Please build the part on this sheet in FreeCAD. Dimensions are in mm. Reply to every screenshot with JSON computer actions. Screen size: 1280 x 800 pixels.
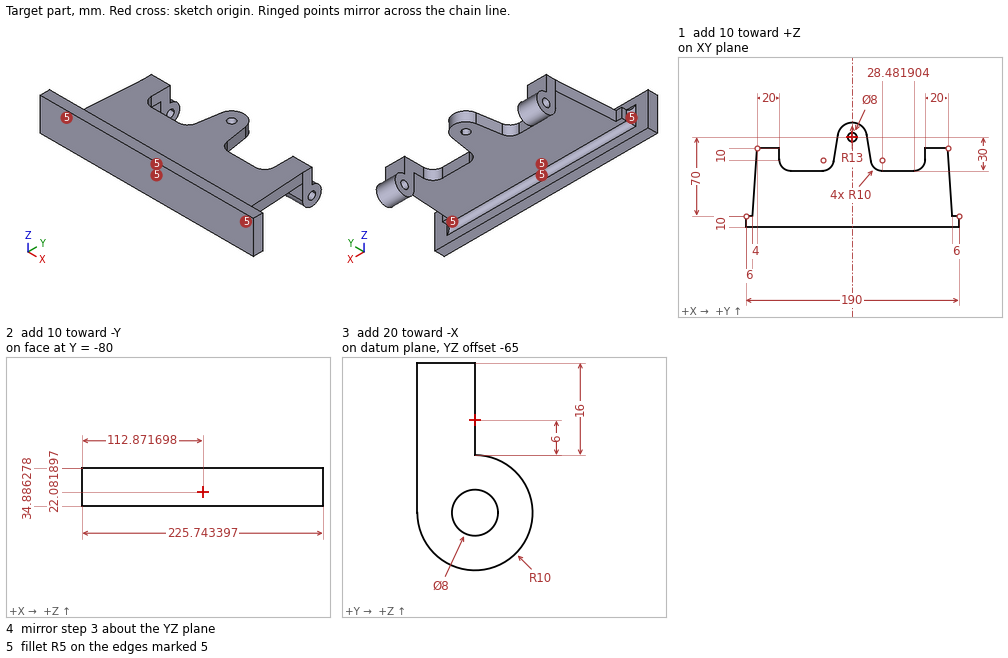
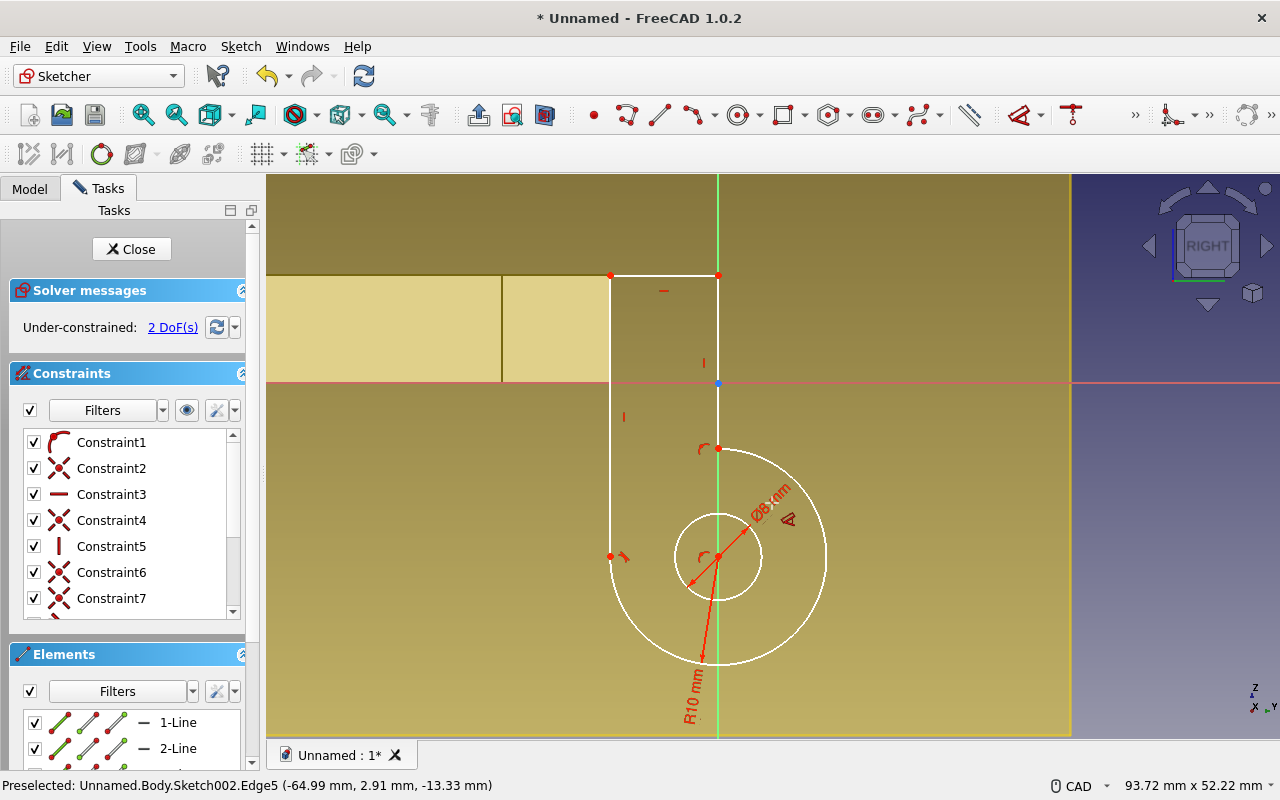
{"action": "left_click", "coordinate": [718, 397]}
{"action": "left_click", "coordinate": [752, 362]}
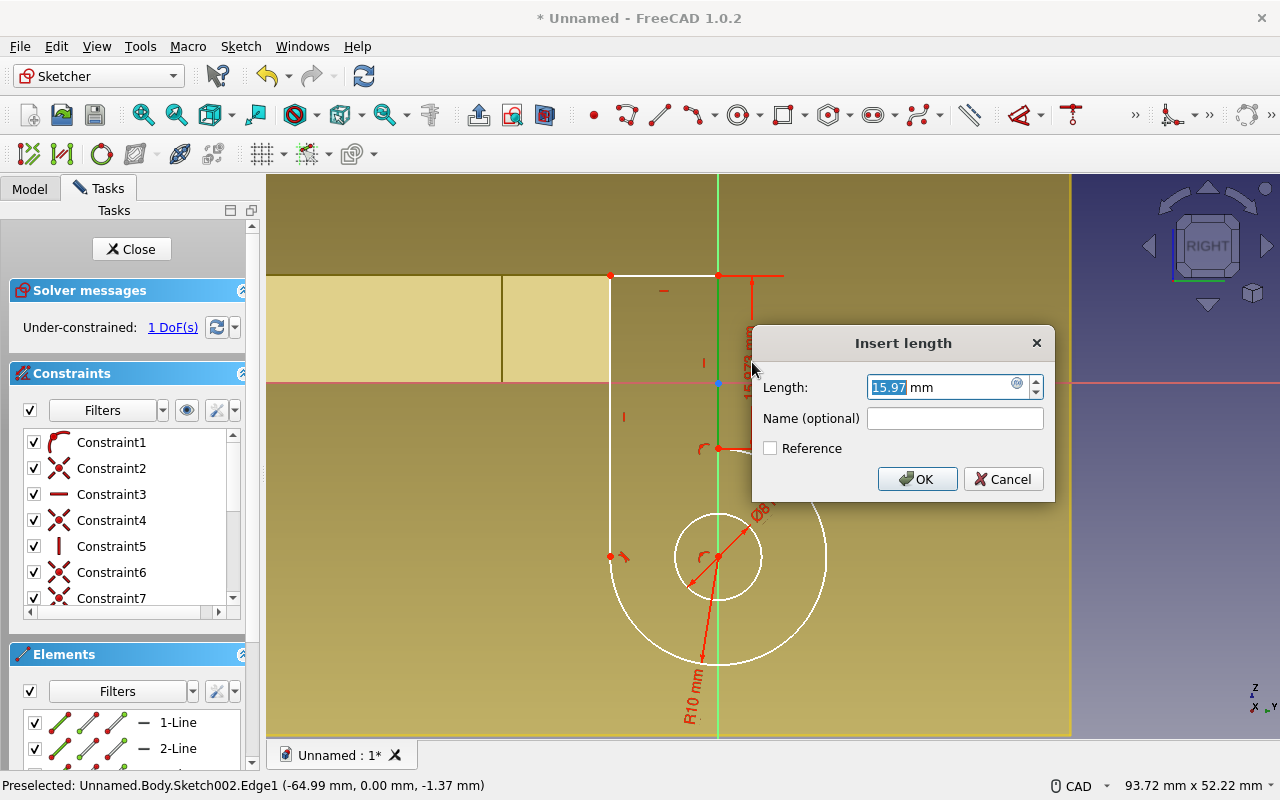
{"action": "type", "text": "16"}
{"action": "key", "text": "Return"}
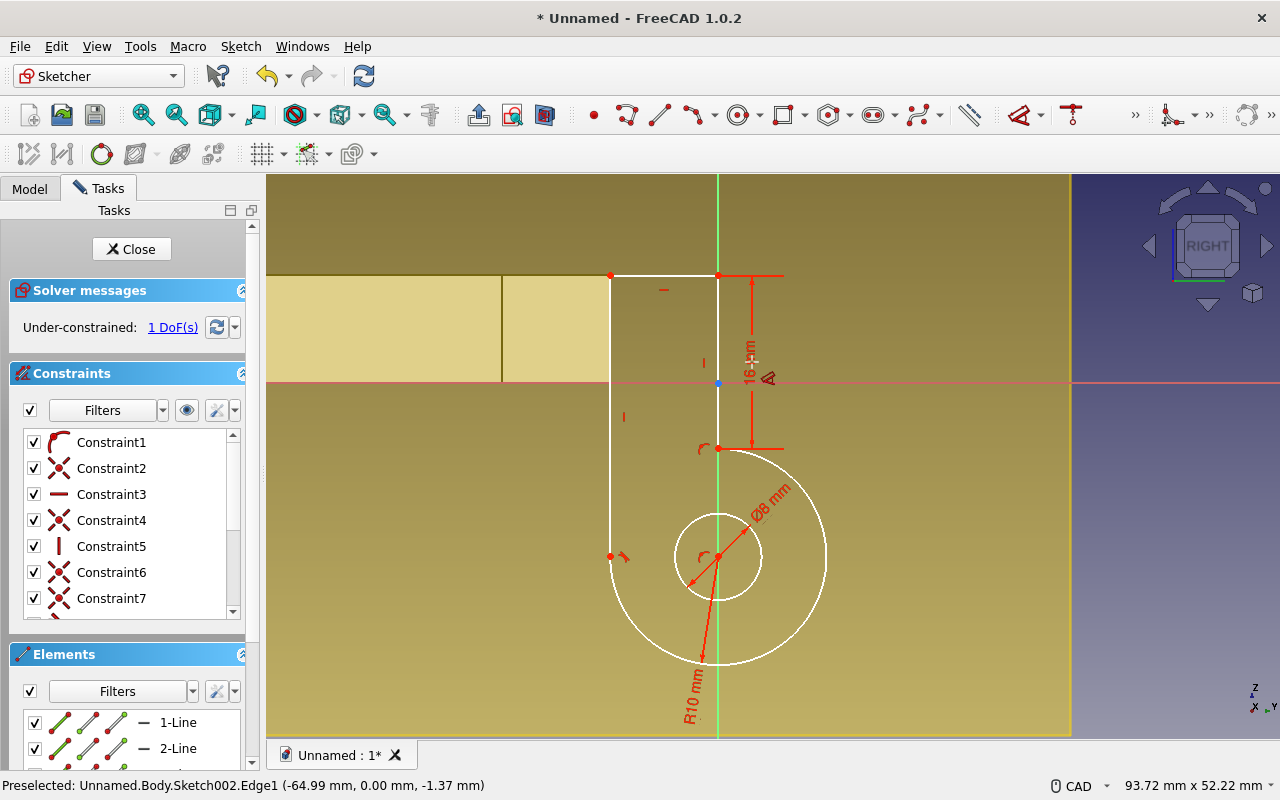
{"action": "left_click", "coordinate": [718, 449]}
{"action": "left_click", "coordinate": [752, 416]}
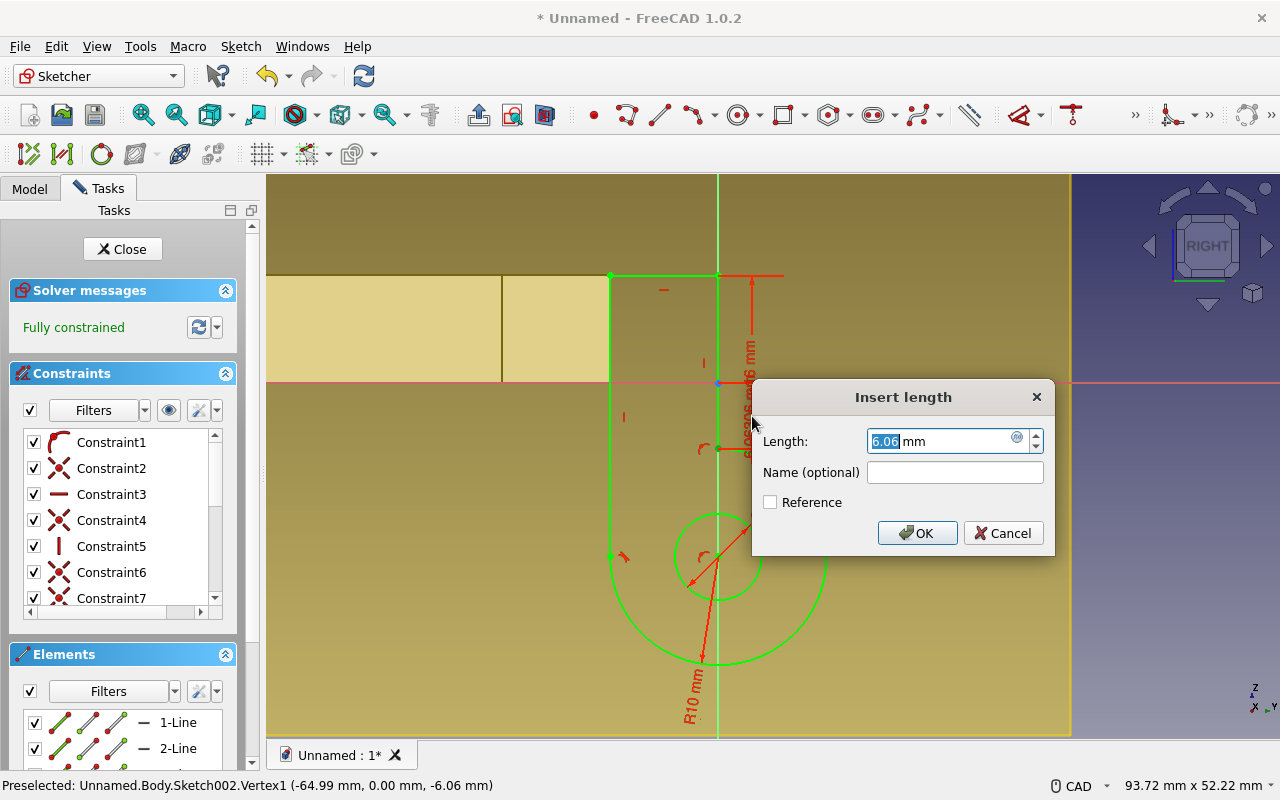
{"action": "type", "text": "6"}
{"action": "key", "text": "Return"}
{"action": "key", "text": "Escape"}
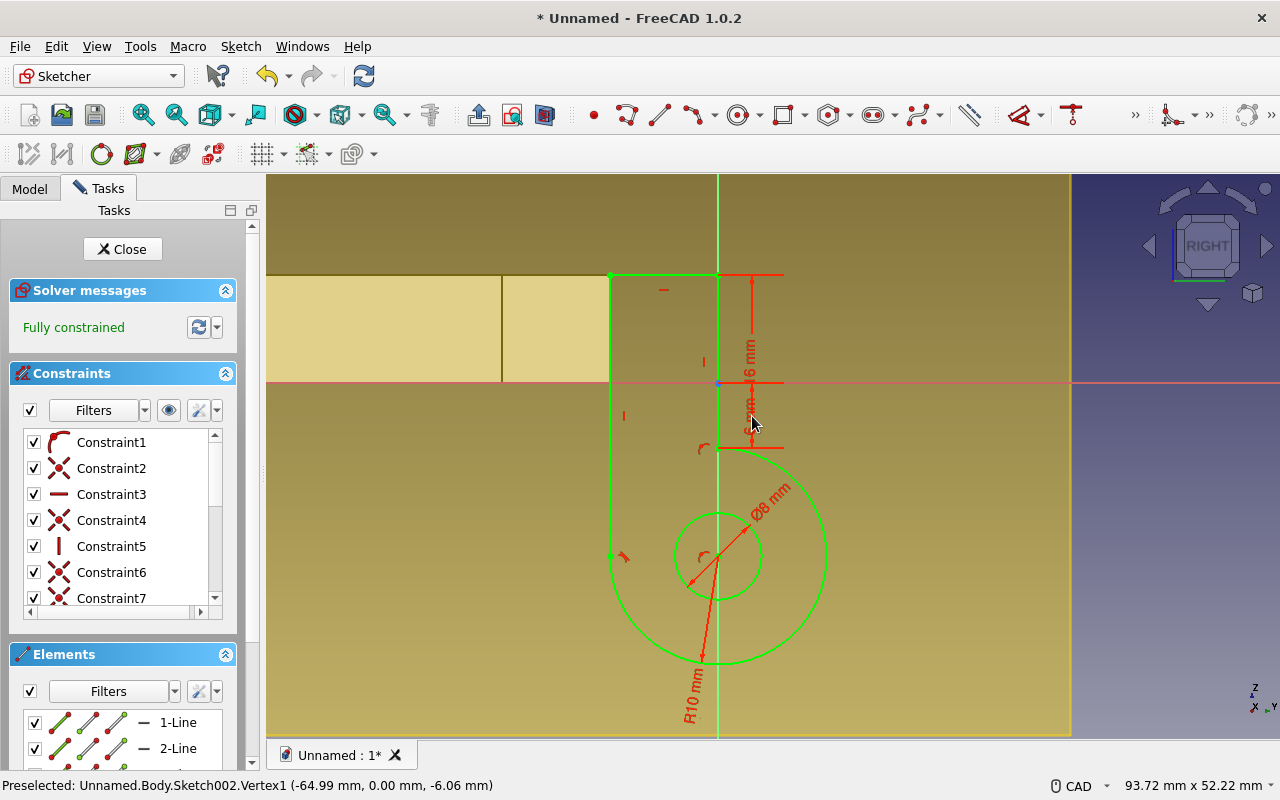
{"action": "left_click", "coordinate": [123, 249]}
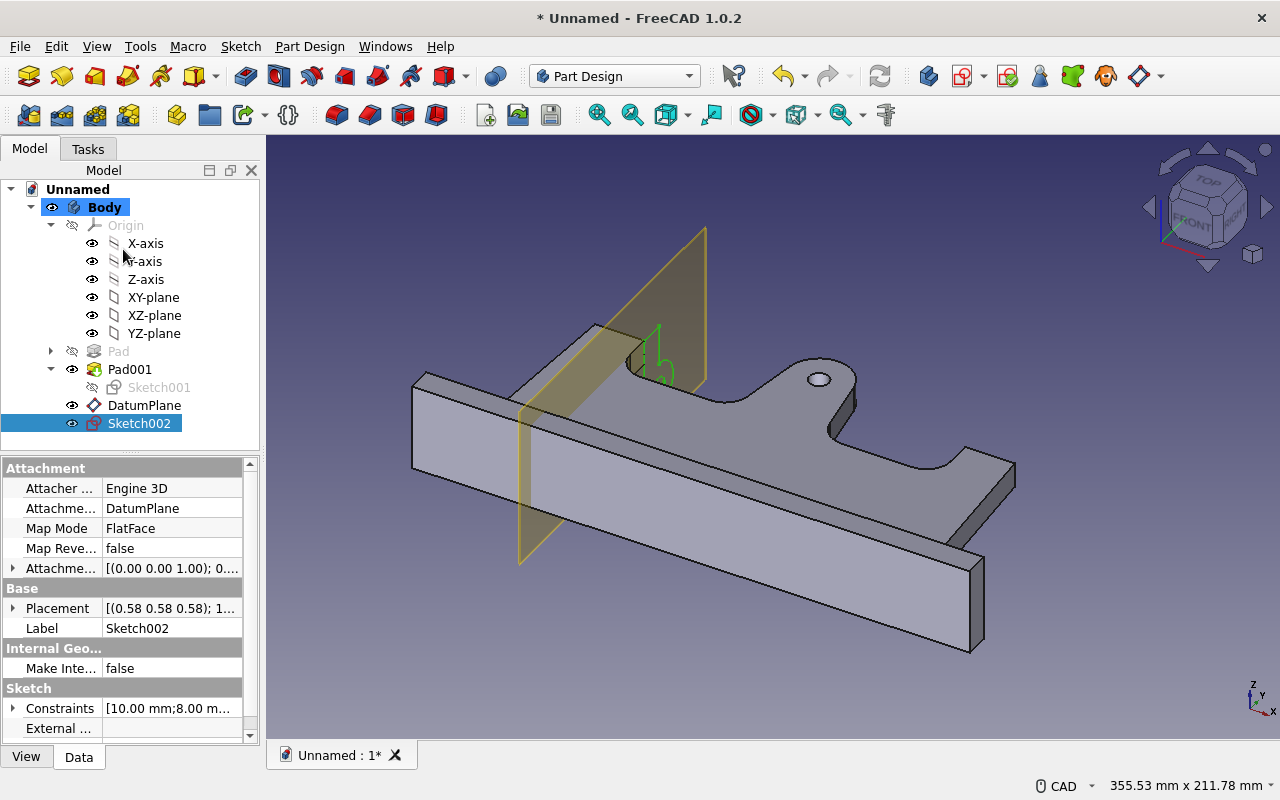
{"action": "left_click", "coordinate": [29, 76]}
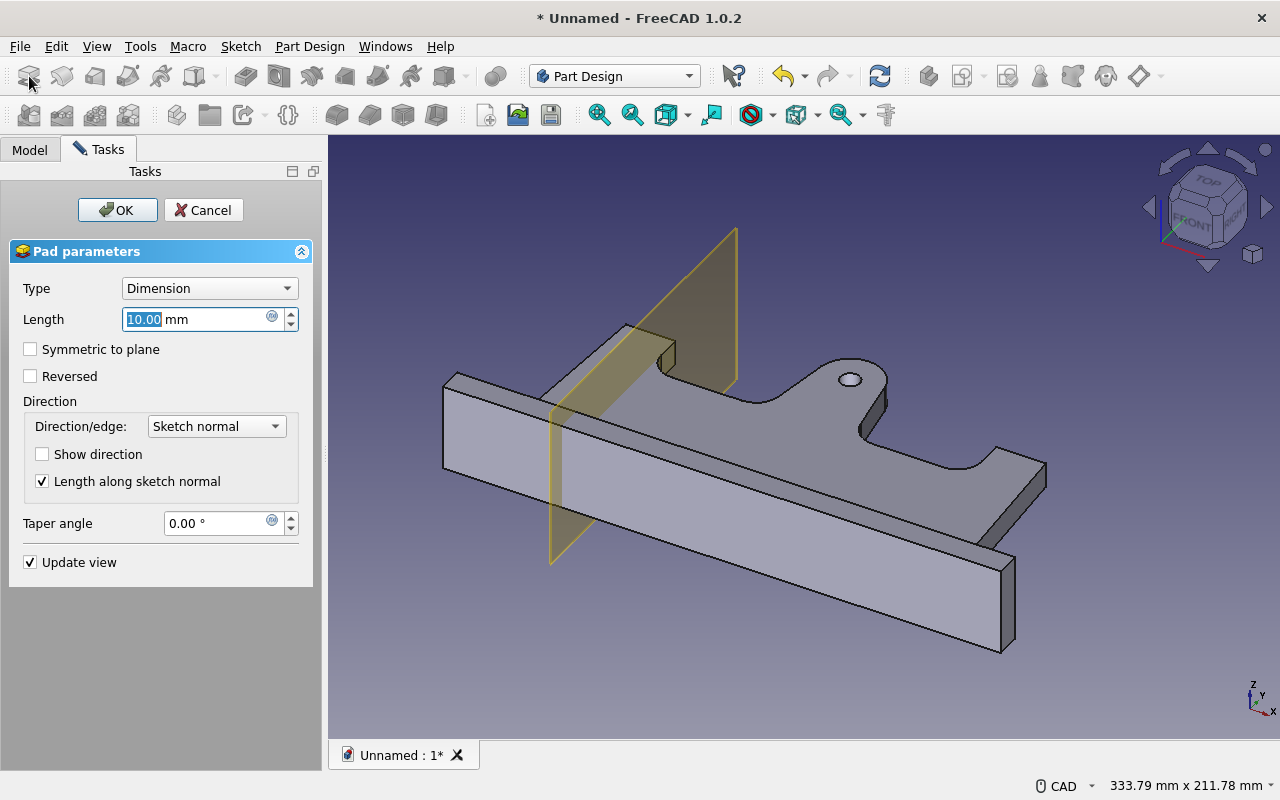
{"action": "type", "text": "20"}
{"action": "key", "text": "Tab"}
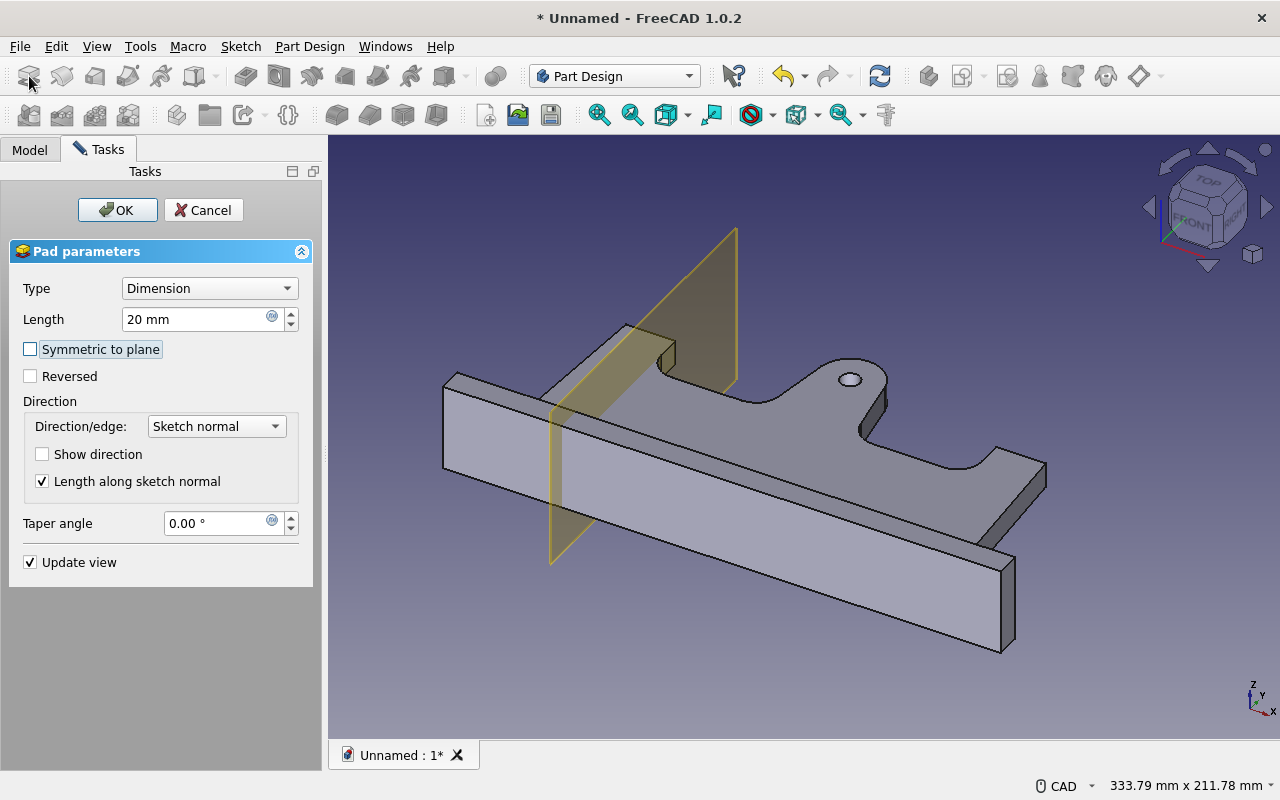
{"action": "left_click", "coordinate": [31, 376]}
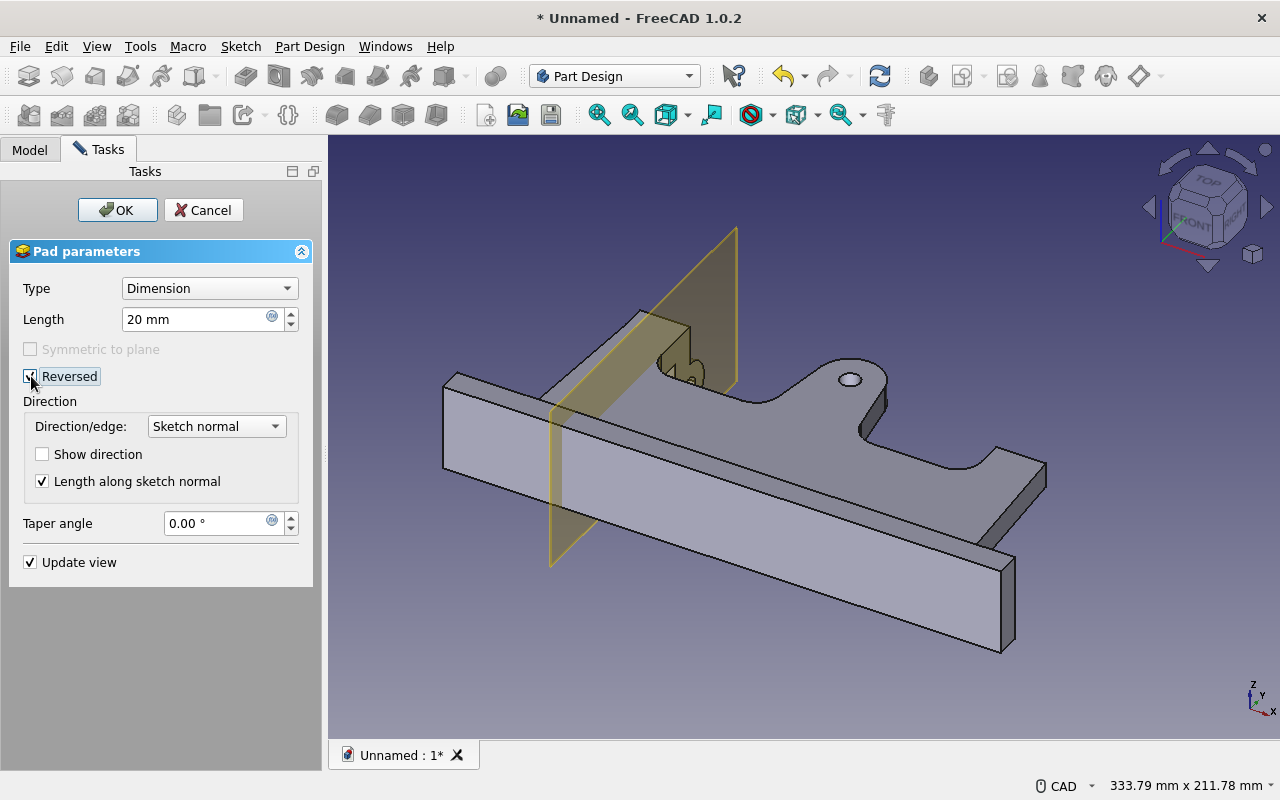
{"action": "left_click", "coordinate": [118, 210]}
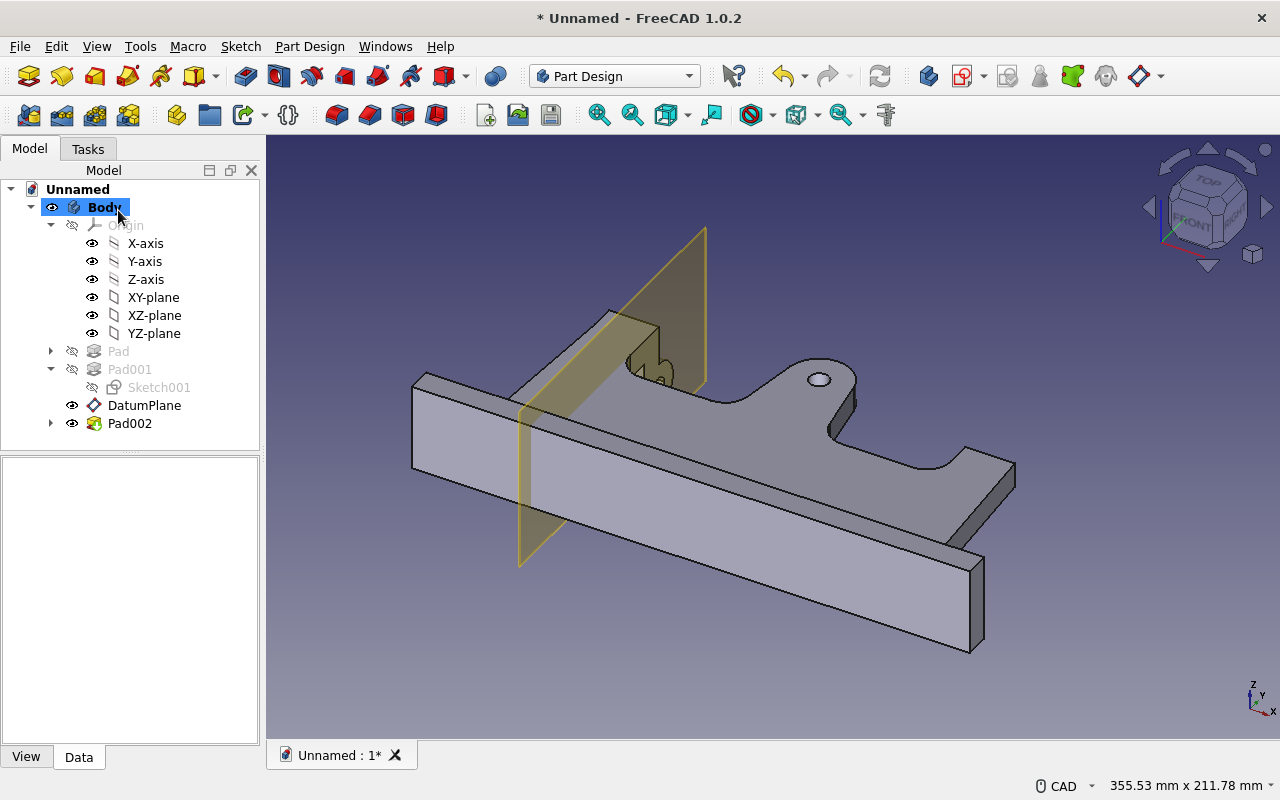
{"action": "left_click", "coordinate": [117, 405]}
{"action": "key", "text": "space"}